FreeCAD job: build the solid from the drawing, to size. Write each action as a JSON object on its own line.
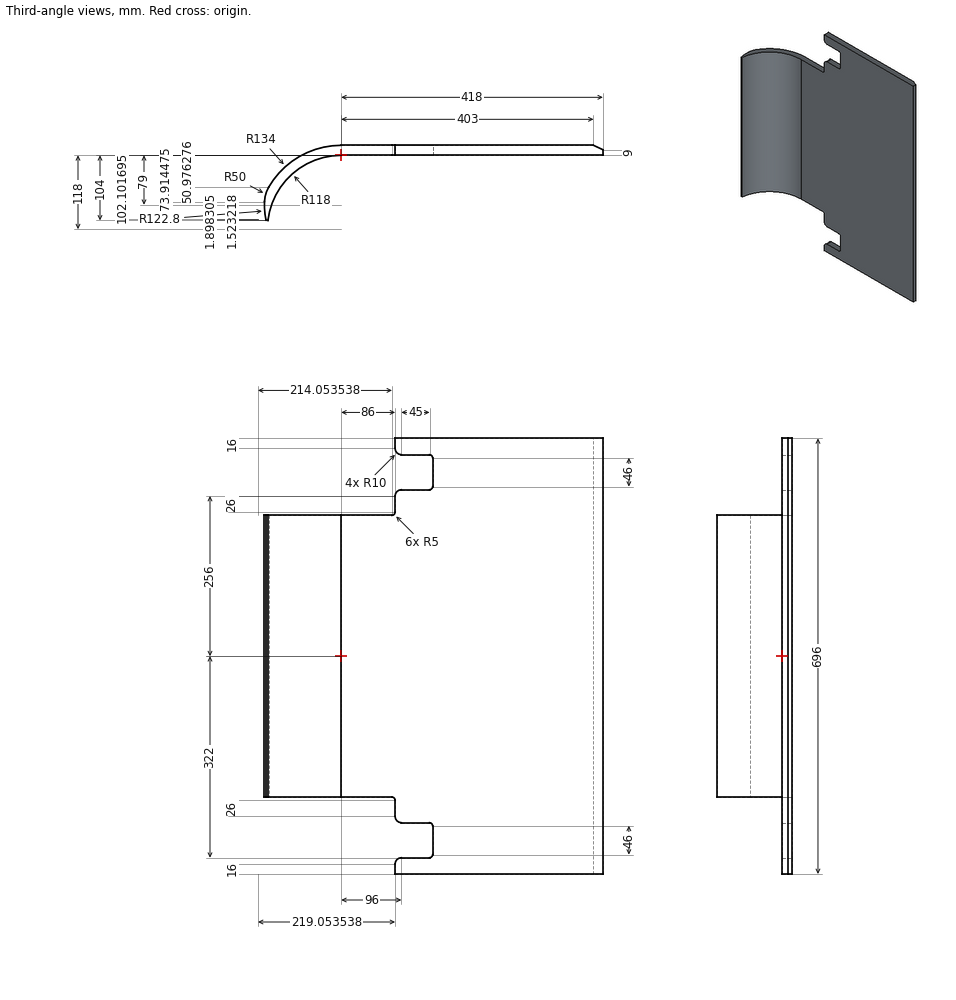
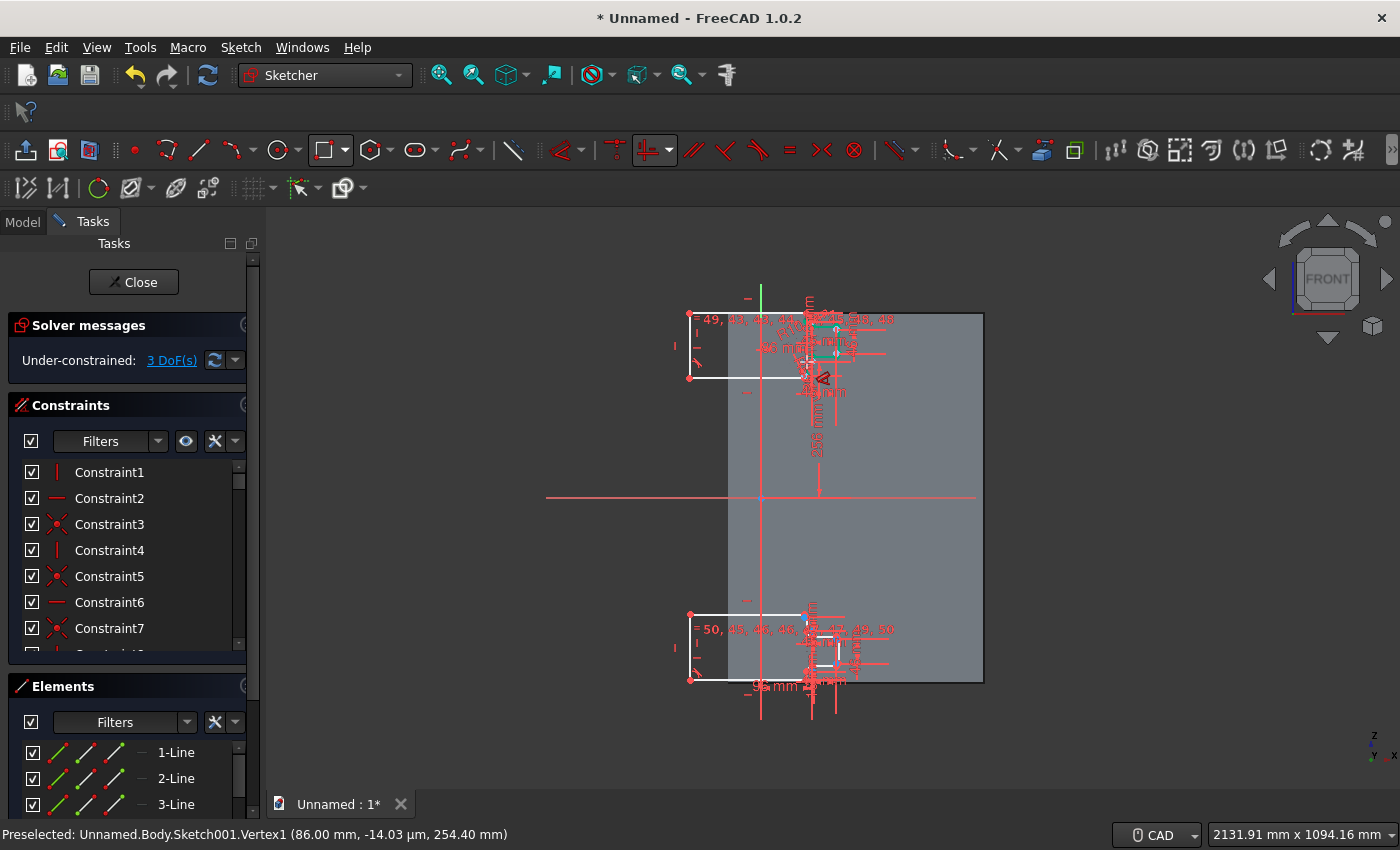
{"action": "scroll", "coordinate": [836, 666], "scroll_direction": "up", "scroll_amount": 8}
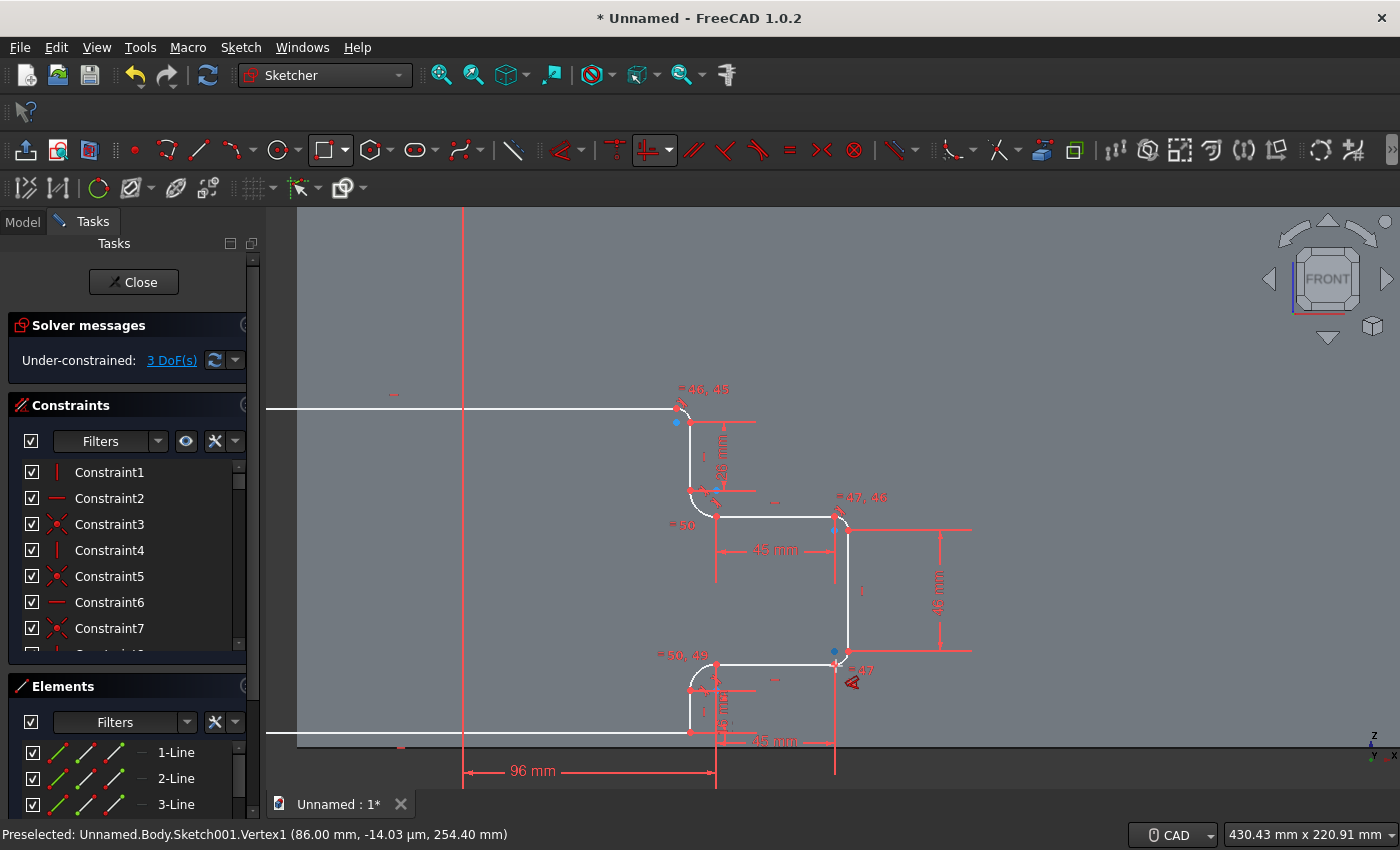
{"action": "left_click", "coordinate": [835, 664]}
{"action": "left_click", "coordinate": [869, 450]}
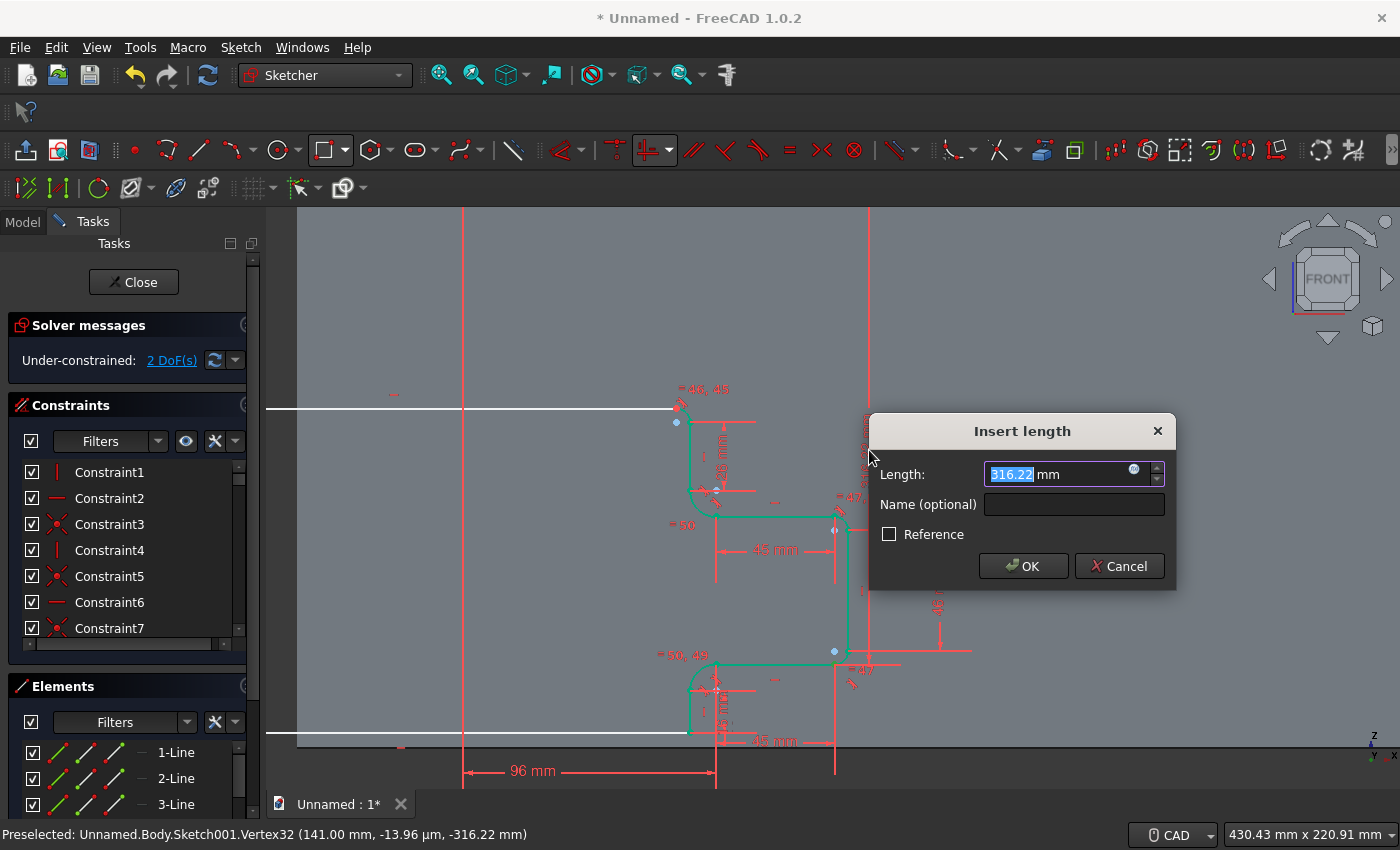
{"action": "type", "text": "322"}
{"action": "key", "text": "Return"}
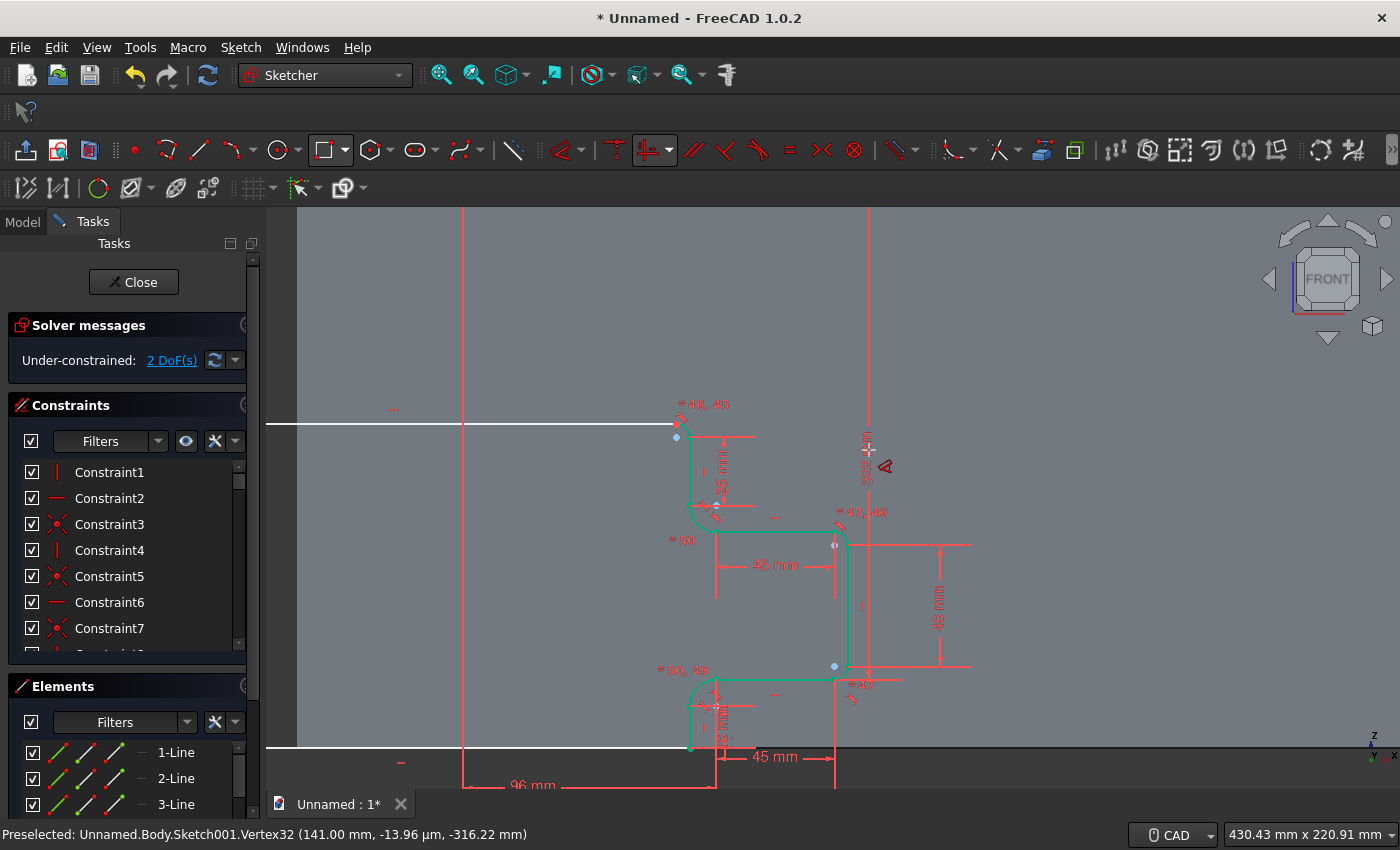
{"action": "scroll", "coordinate": [836, 667], "scroll_direction": "down", "scroll_amount": 8}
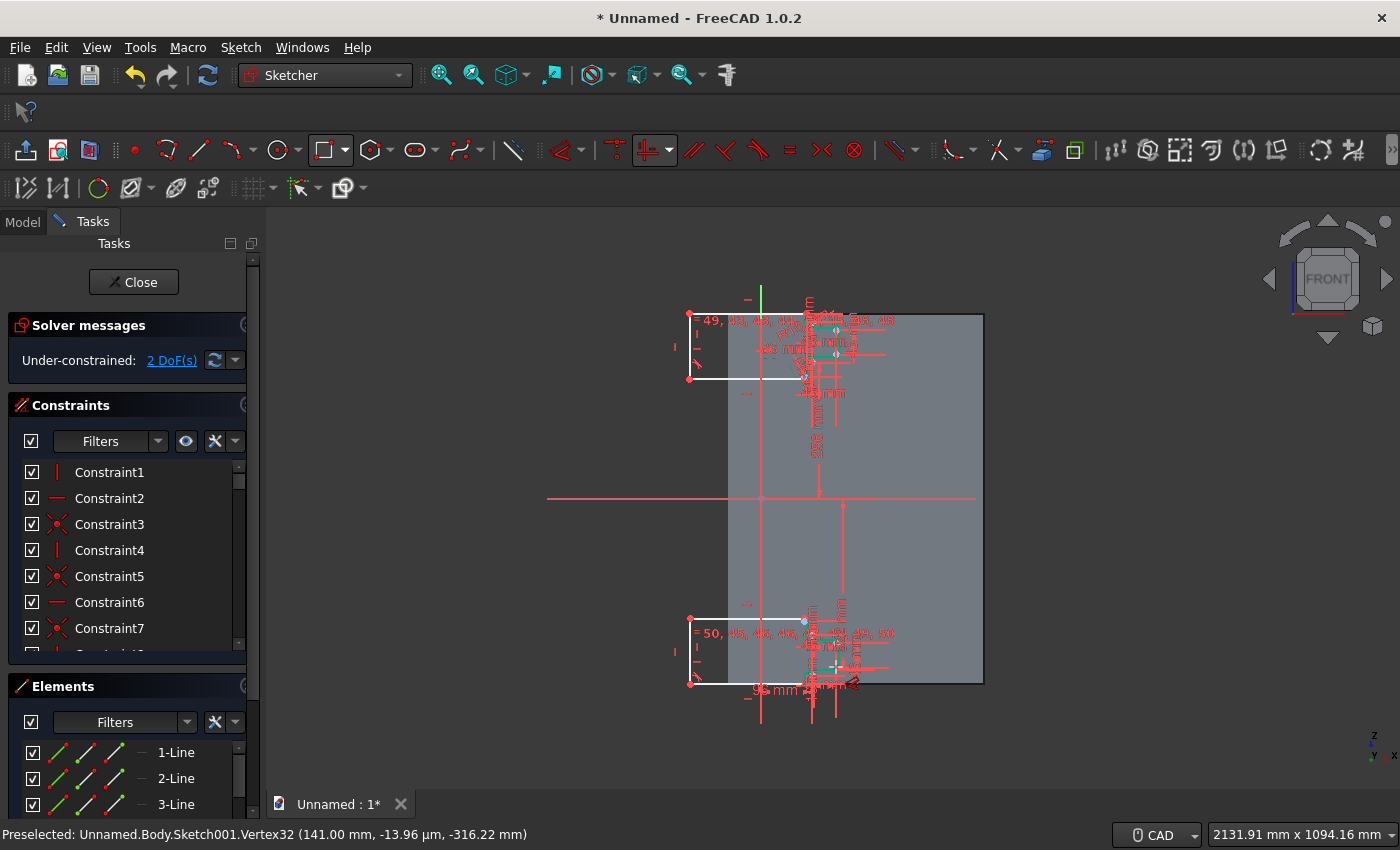
{"action": "scroll", "coordinate": [770, 379], "scroll_direction": "up", "scroll_amount": 3}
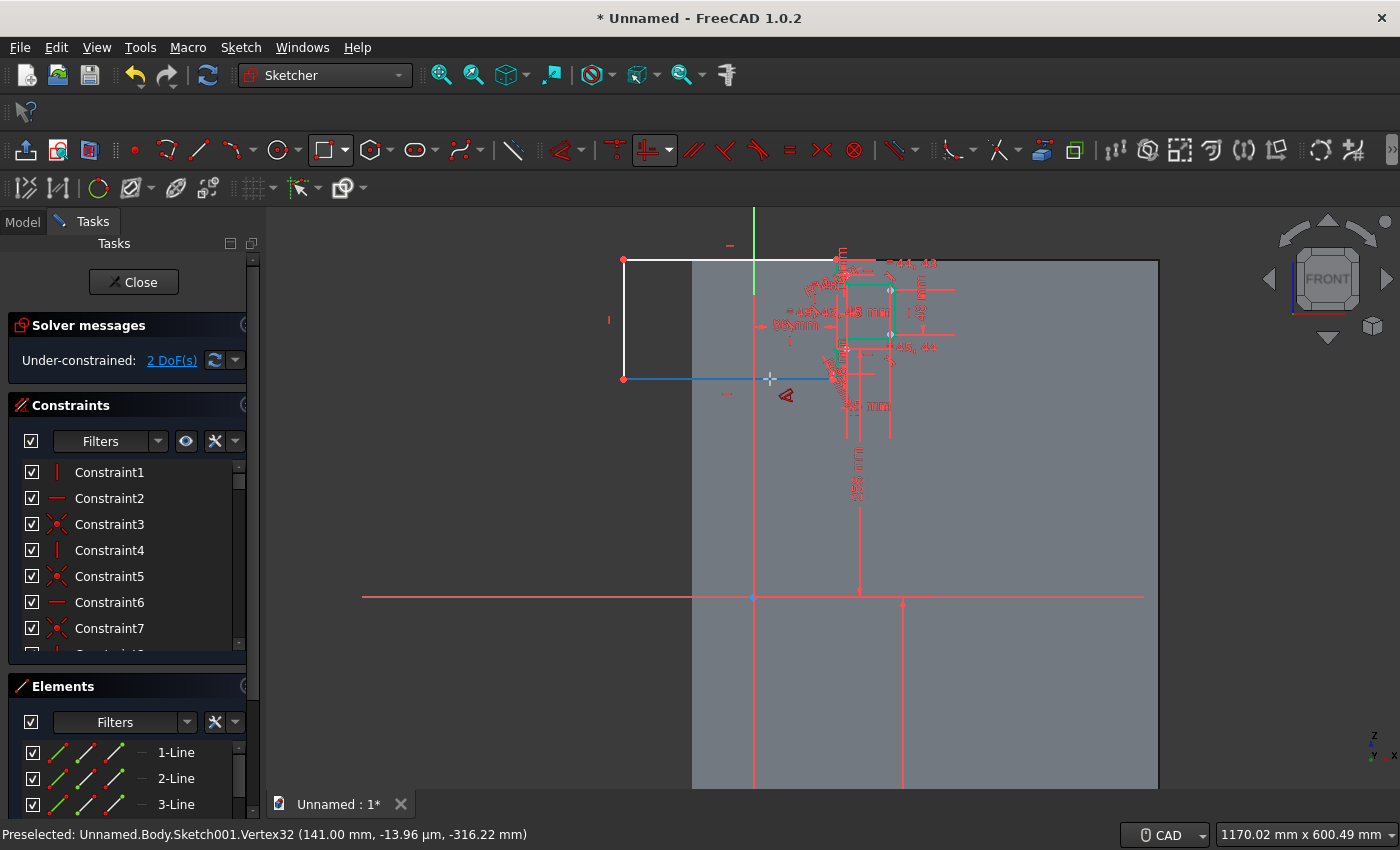
{"action": "left_click", "coordinate": [770, 379]}
{"action": "left_click", "coordinate": [680, 345]}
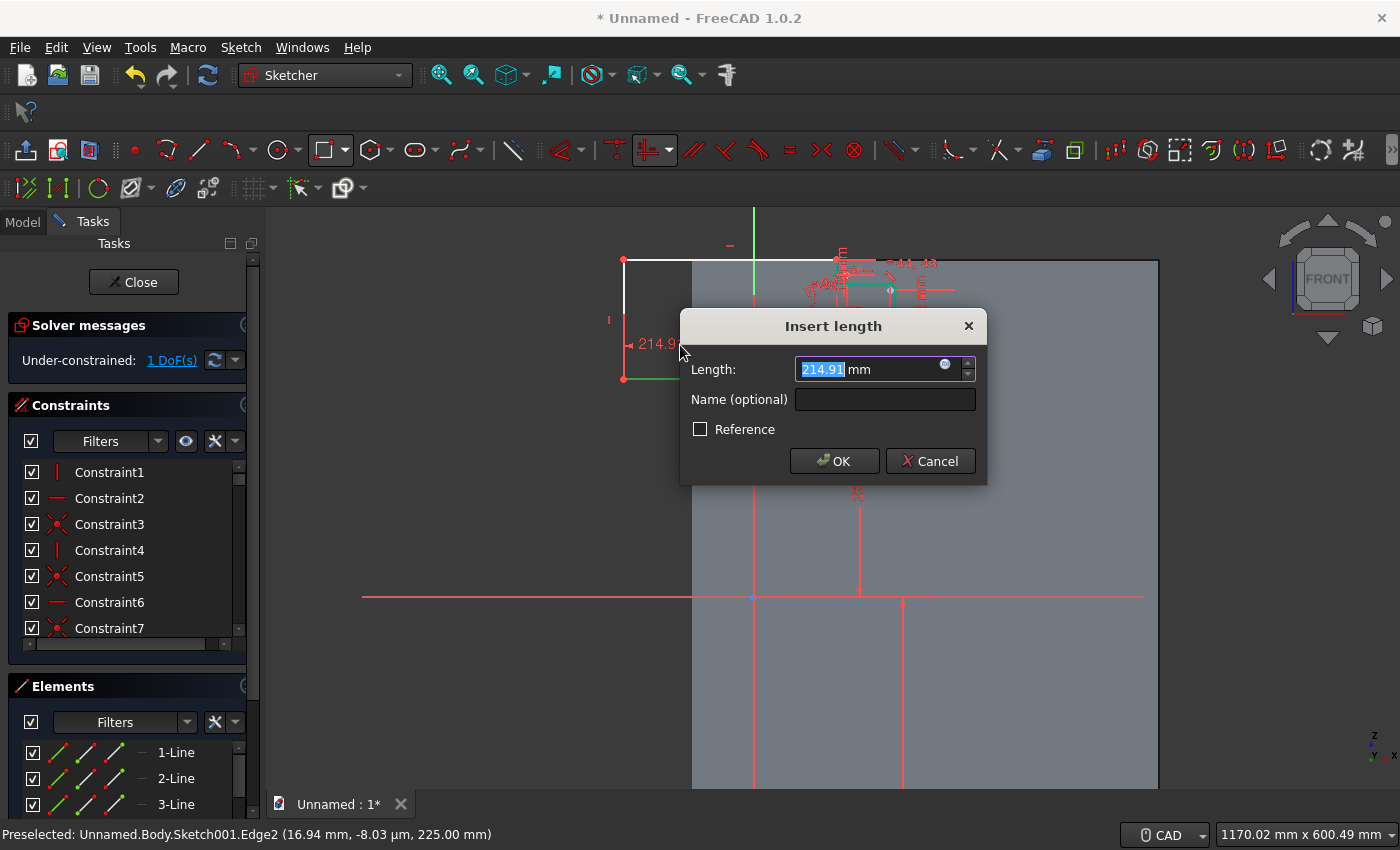
{"action": "type", "text": "214.053538"}
{"action": "key", "text": "Return"}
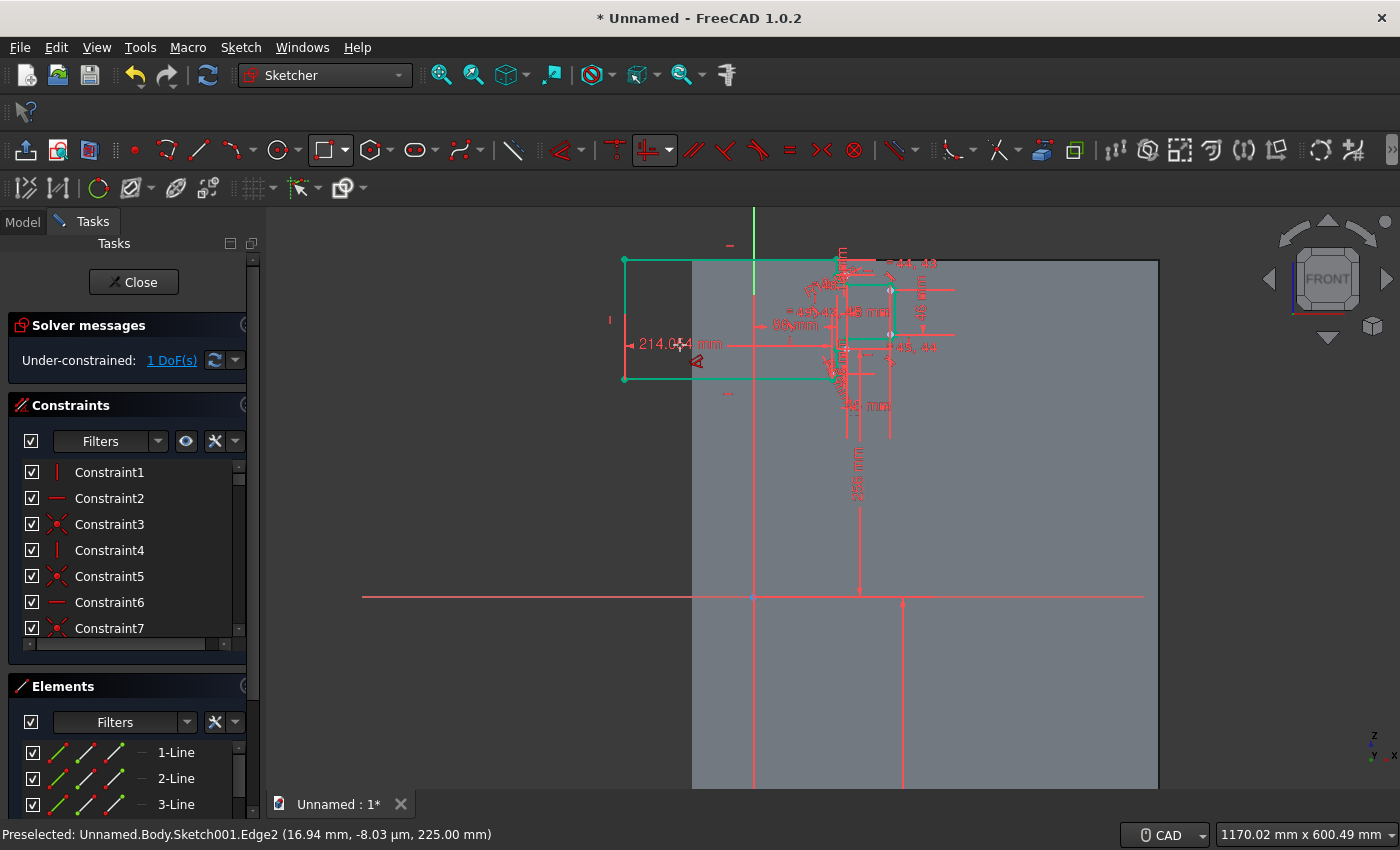
{"action": "scroll", "coordinate": [770, 377], "scroll_direction": "down", "scroll_amount": 3}